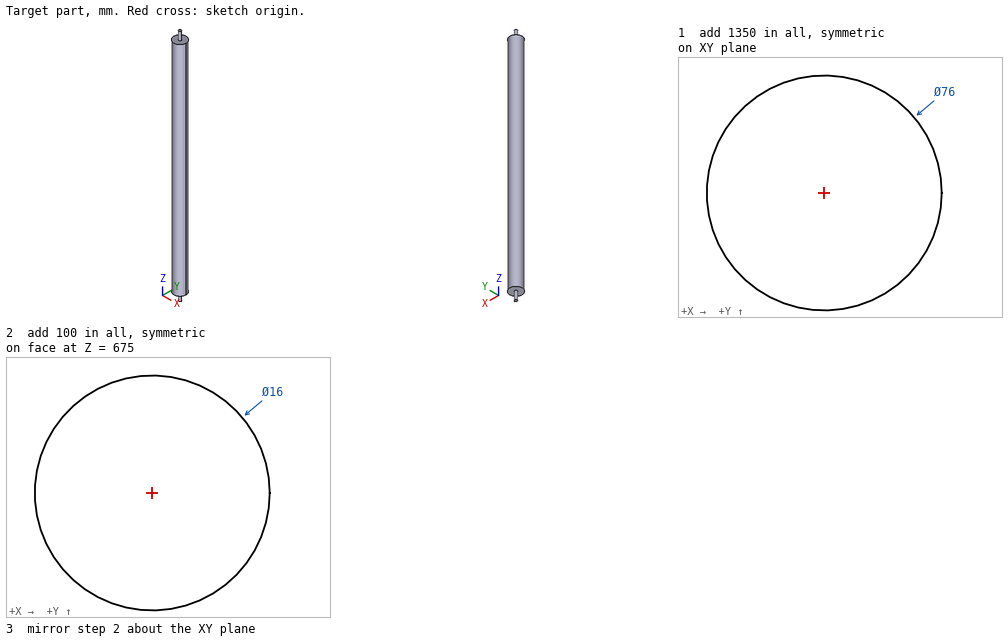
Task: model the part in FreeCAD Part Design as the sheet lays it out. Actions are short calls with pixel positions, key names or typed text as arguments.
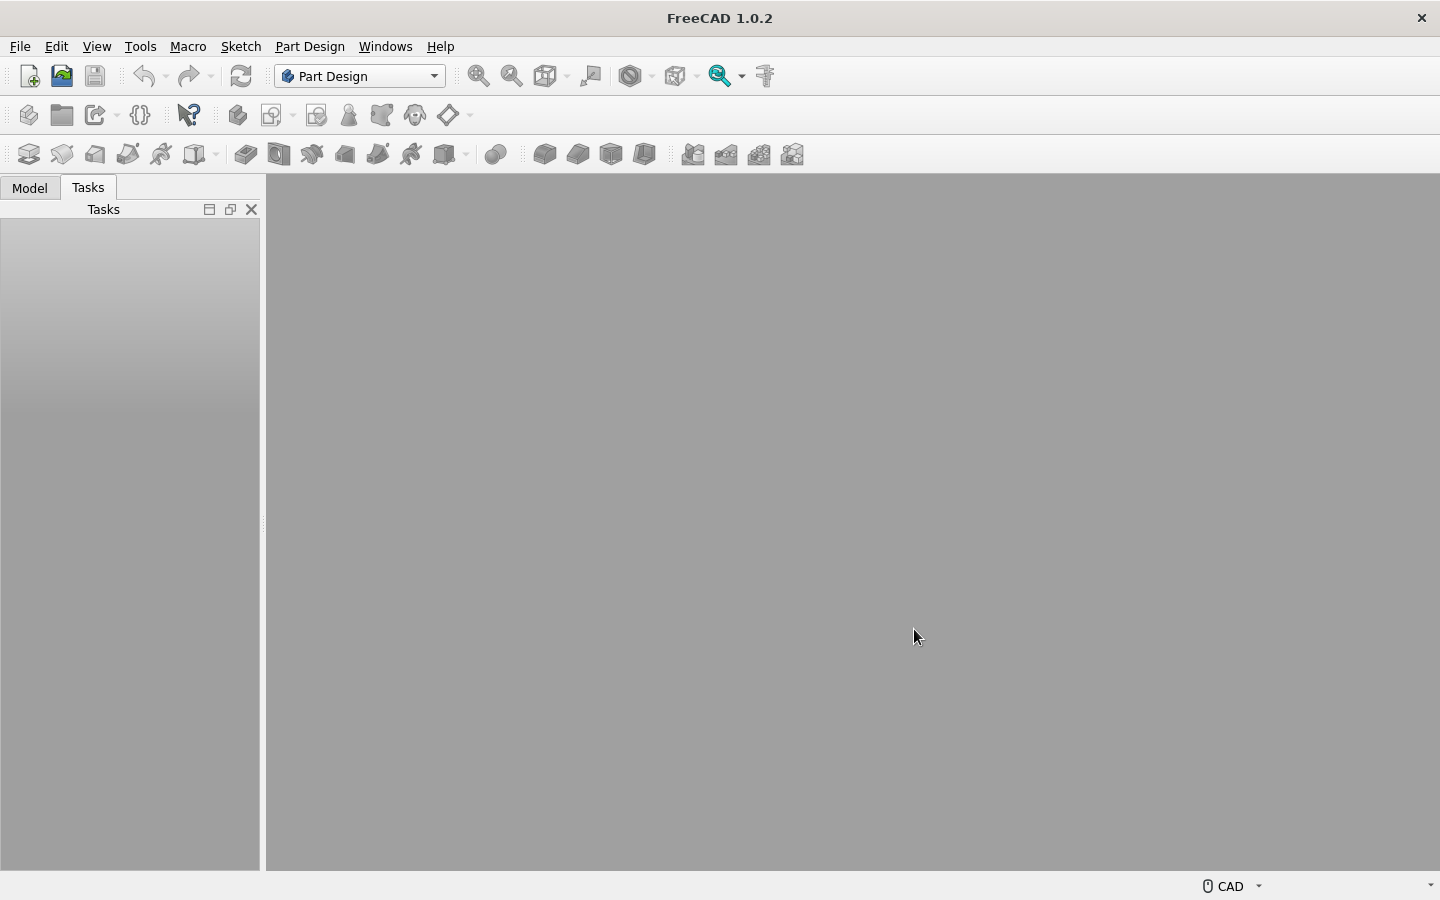
click(29, 76)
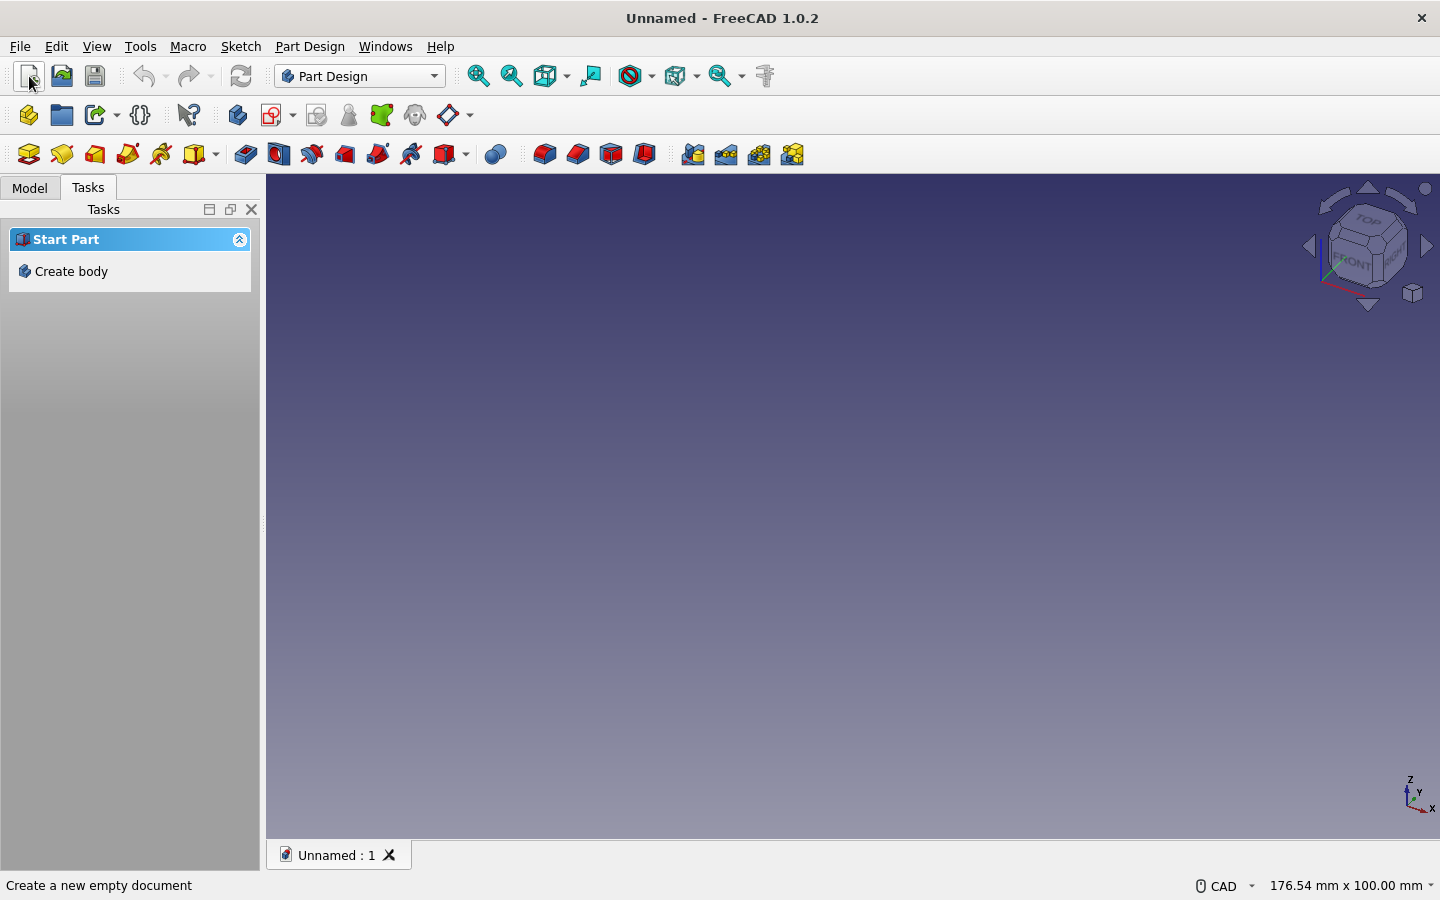
click(270, 116)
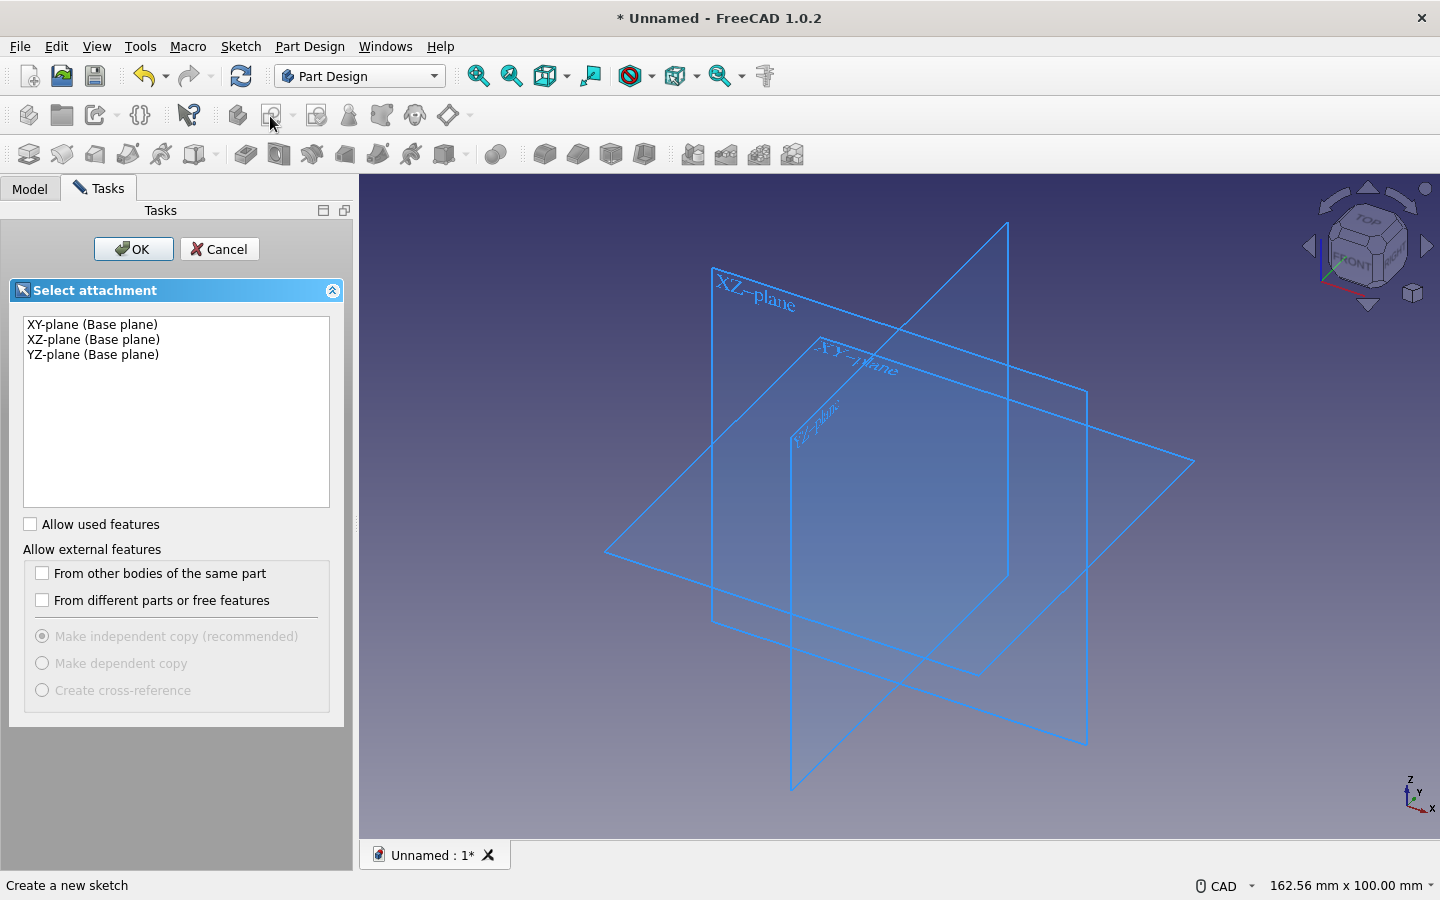
click(84, 324)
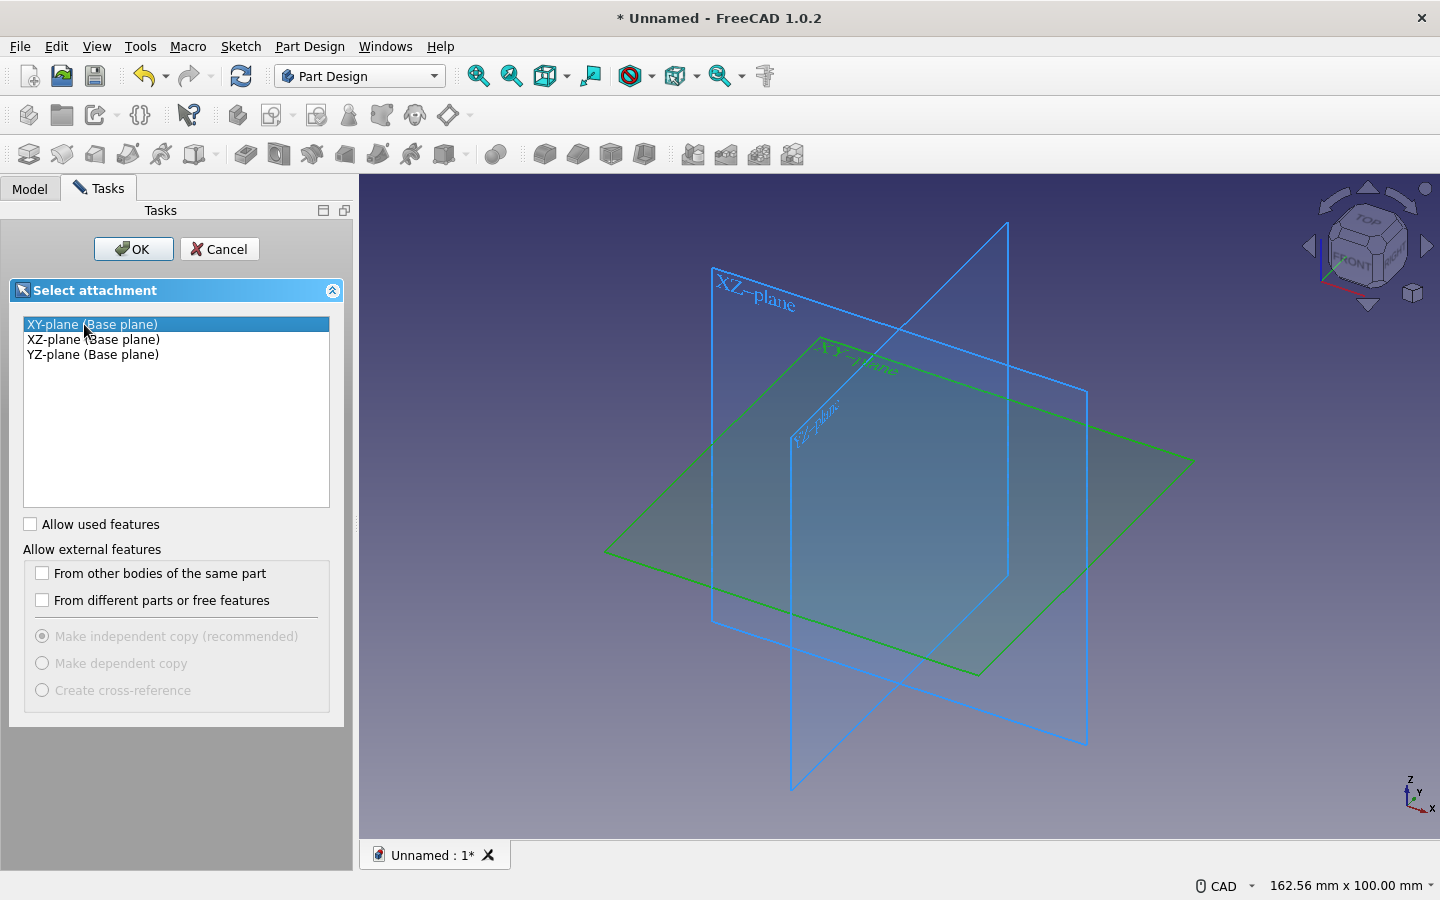
click(134, 249)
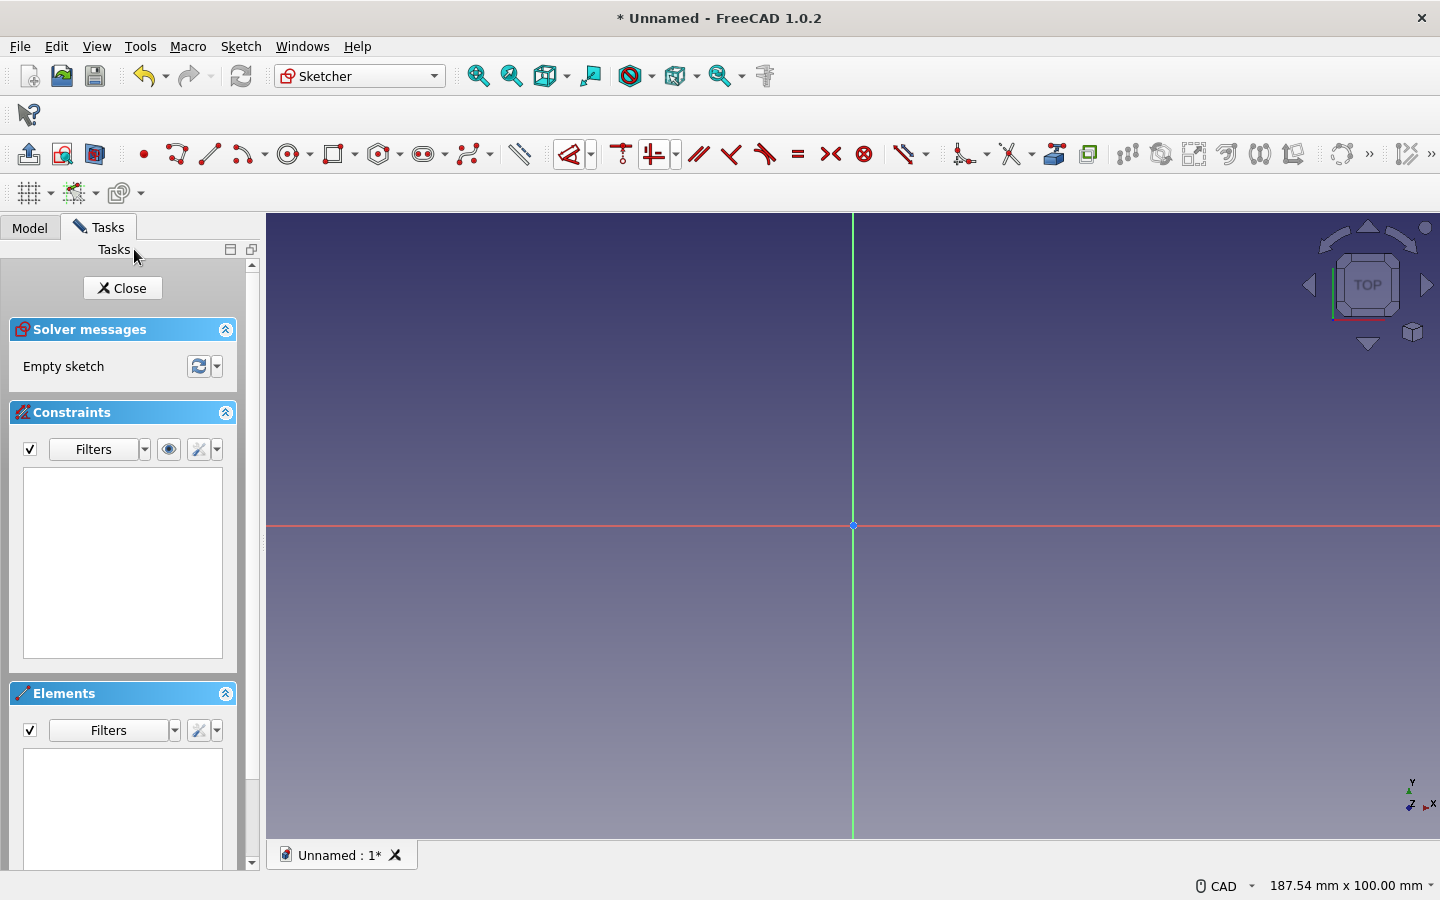
click(288, 154)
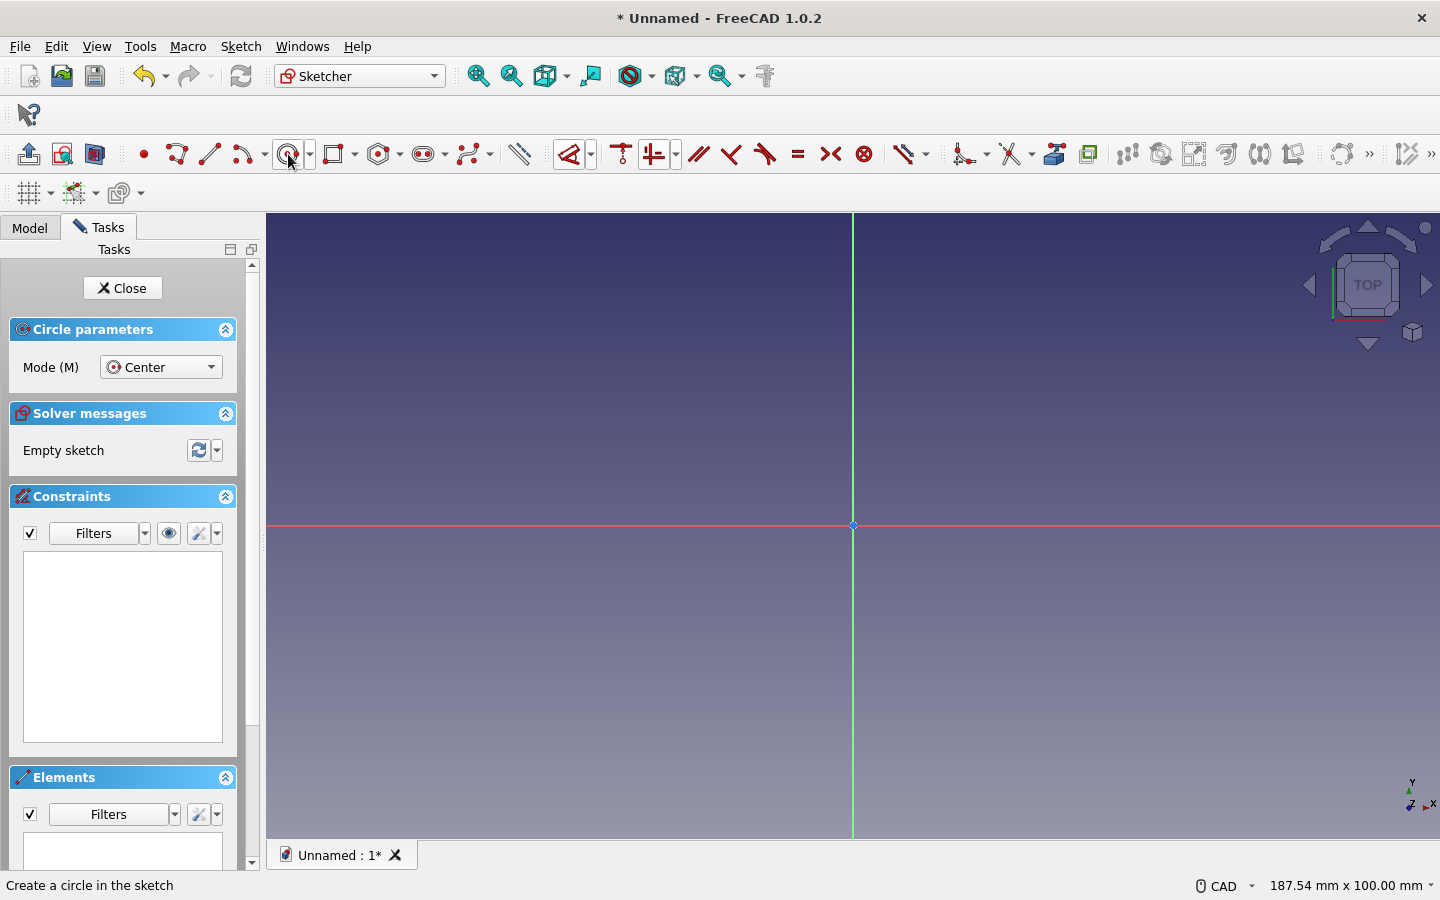
click(853, 526)
click(1021, 358)
key(Escape)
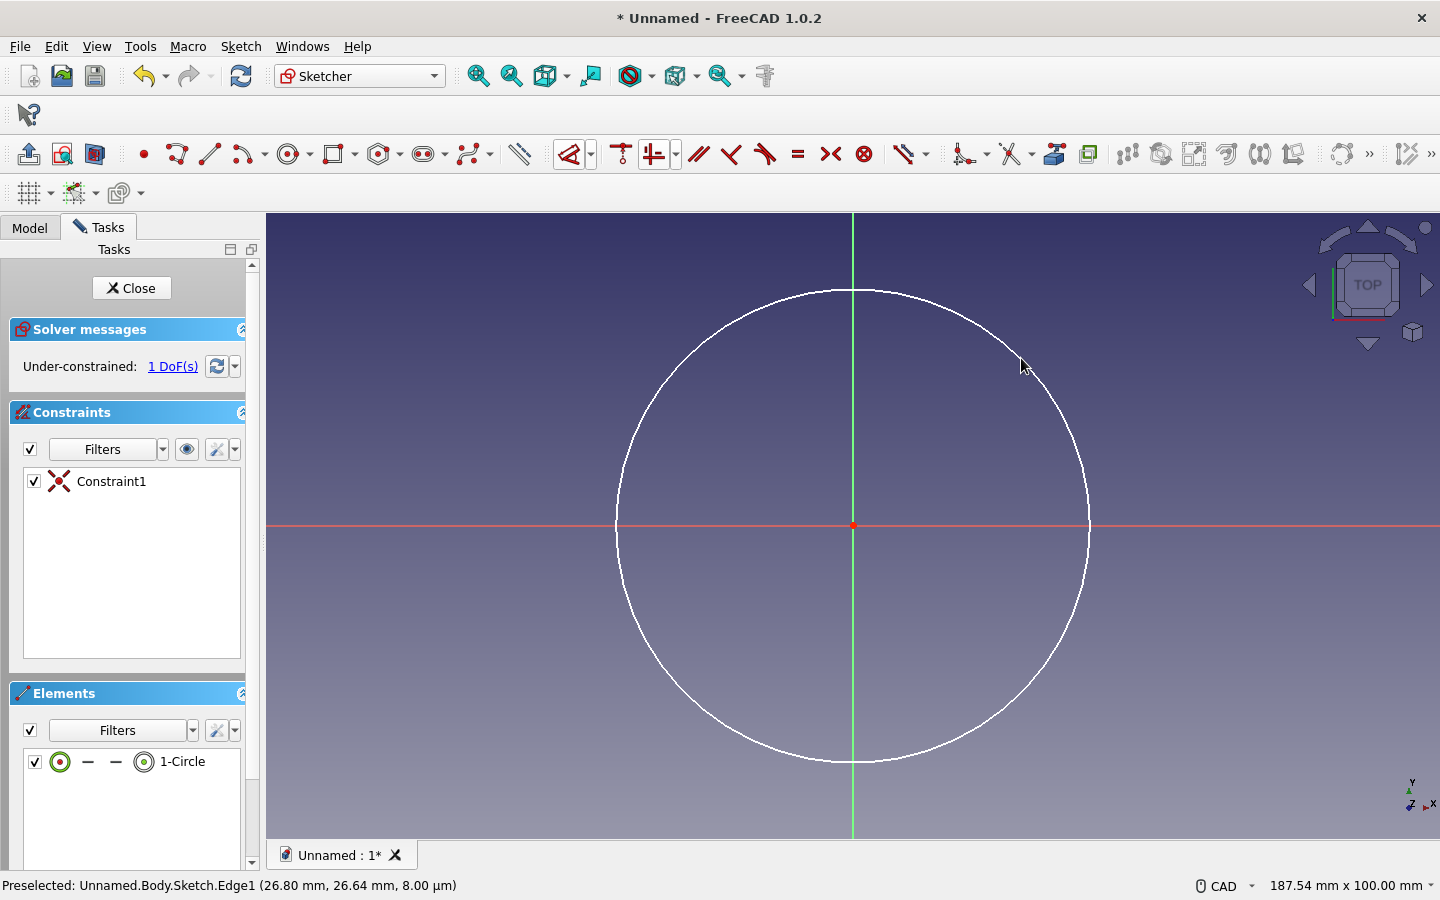
click(568, 154)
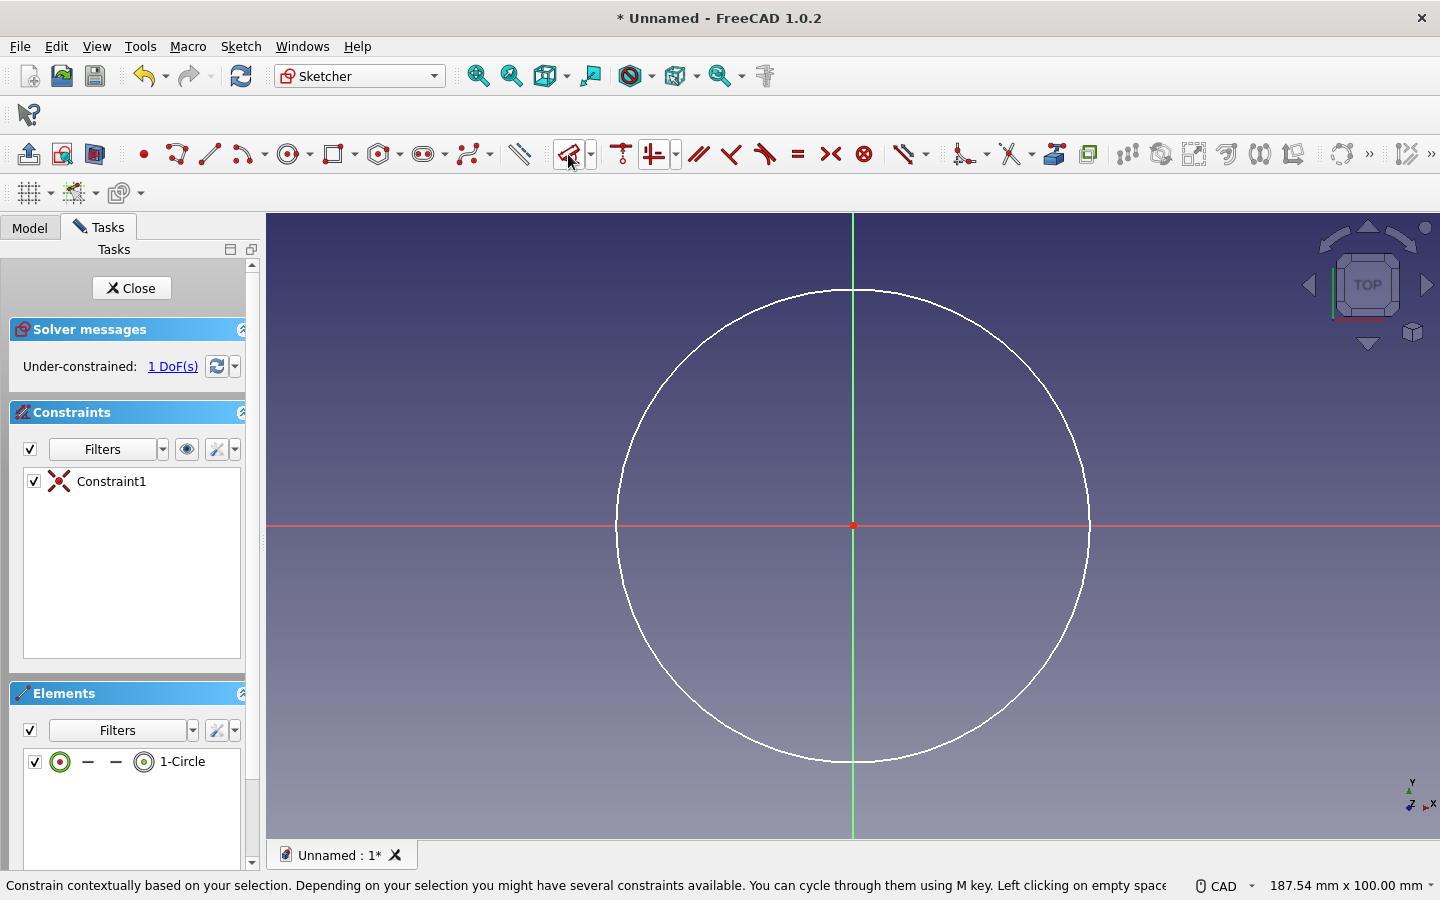
click(1020, 358)
click(1043, 335)